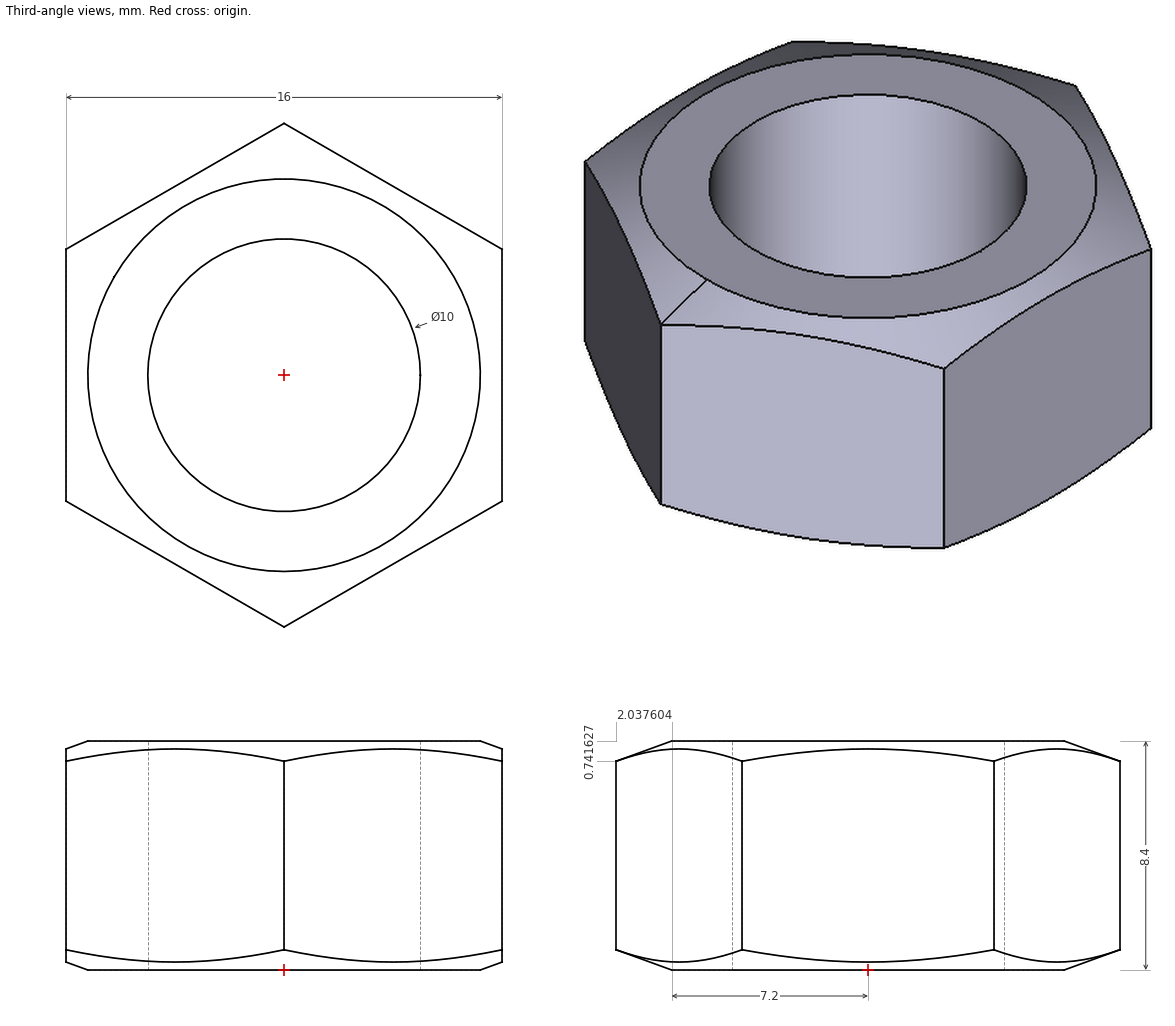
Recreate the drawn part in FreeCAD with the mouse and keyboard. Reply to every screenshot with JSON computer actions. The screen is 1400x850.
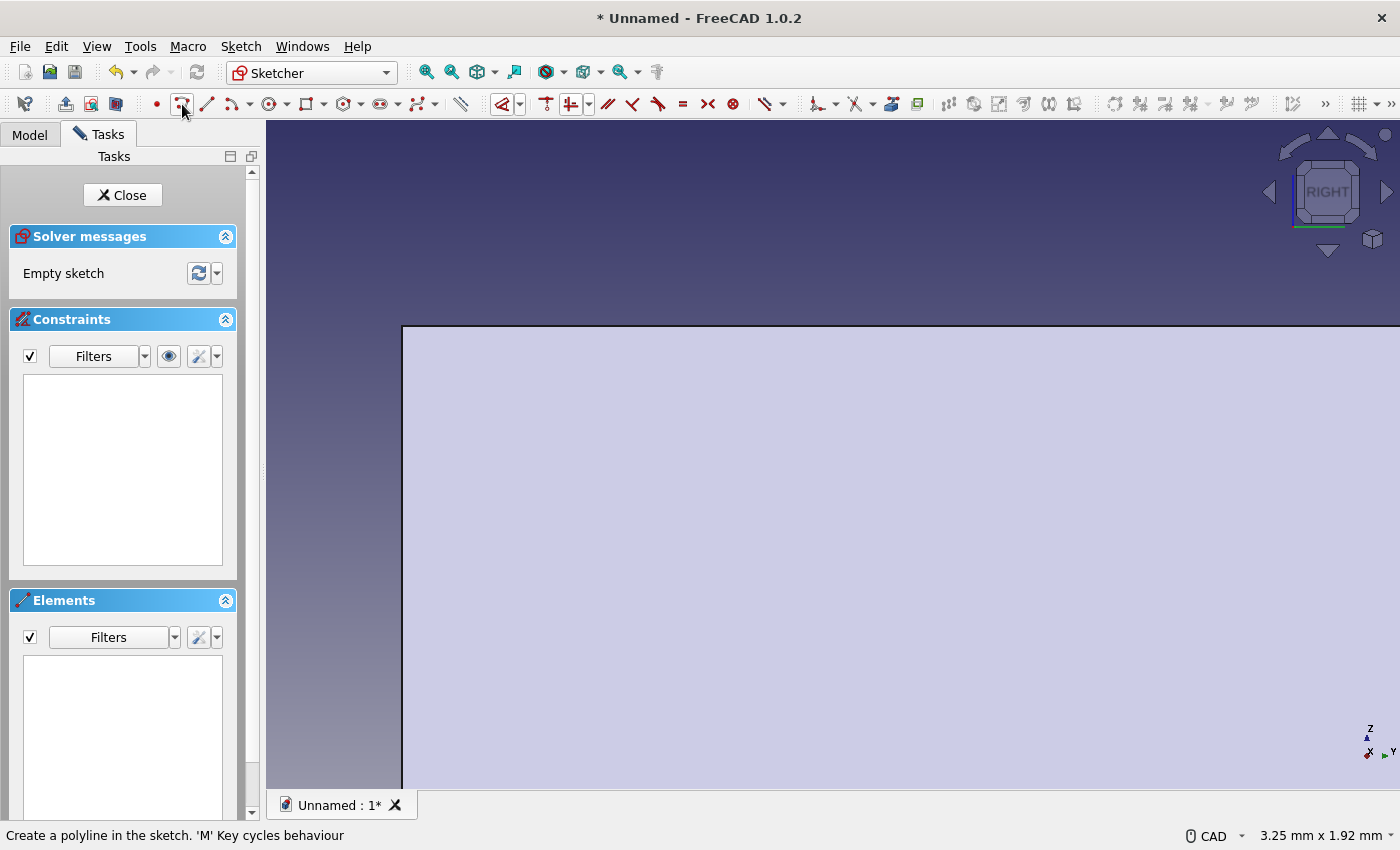
{"action": "left_click", "coordinate": [1112, 326]}
{"action": "left_click", "coordinate": [402, 326]}
{"action": "left_click", "coordinate": [402, 585]}
{"action": "left_click", "coordinate": [1112, 327]}
{"action": "key", "text": "Escape"}
{"action": "key", "text": "Escape"}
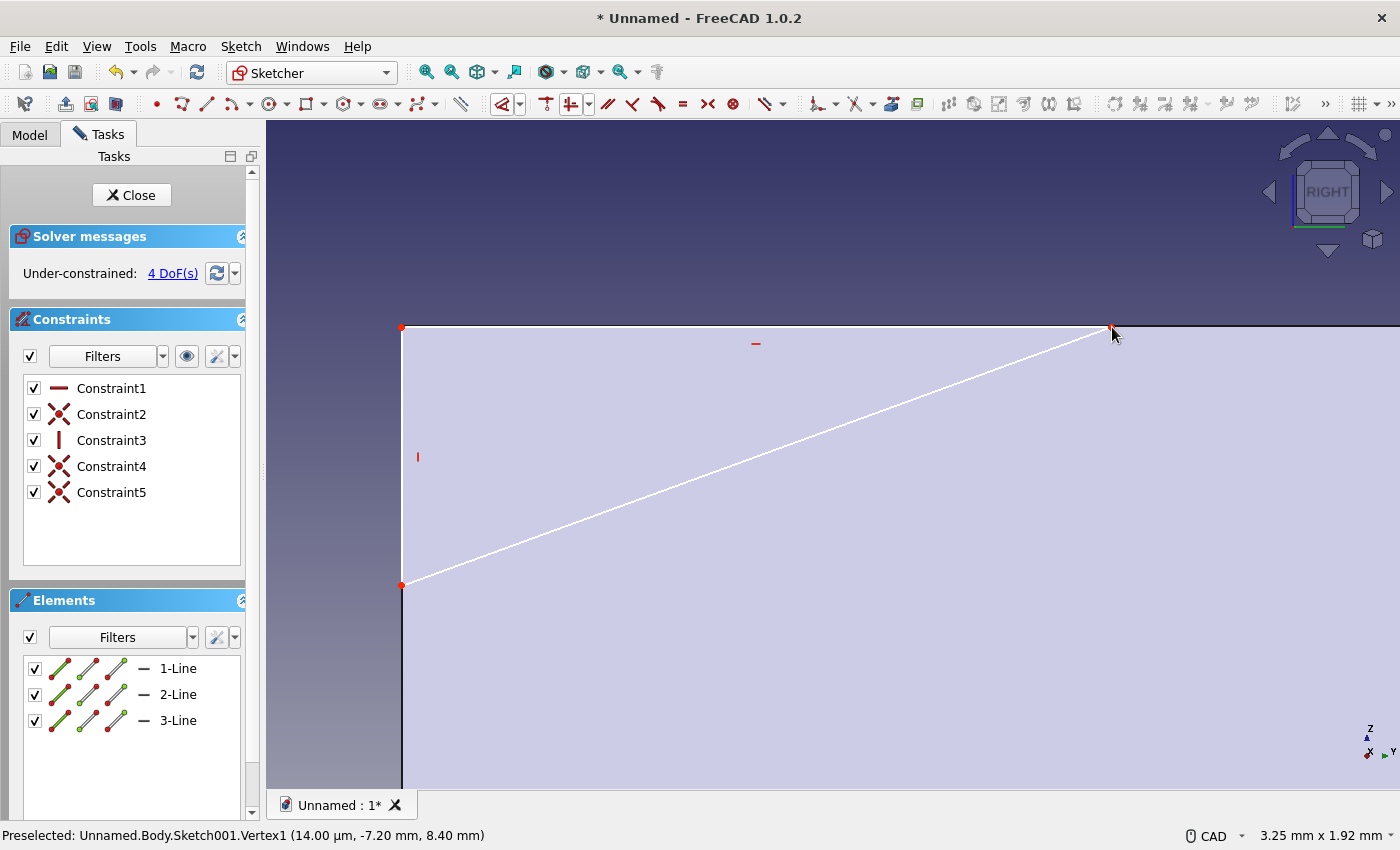
{"action": "left_click", "coordinate": [1112, 327]}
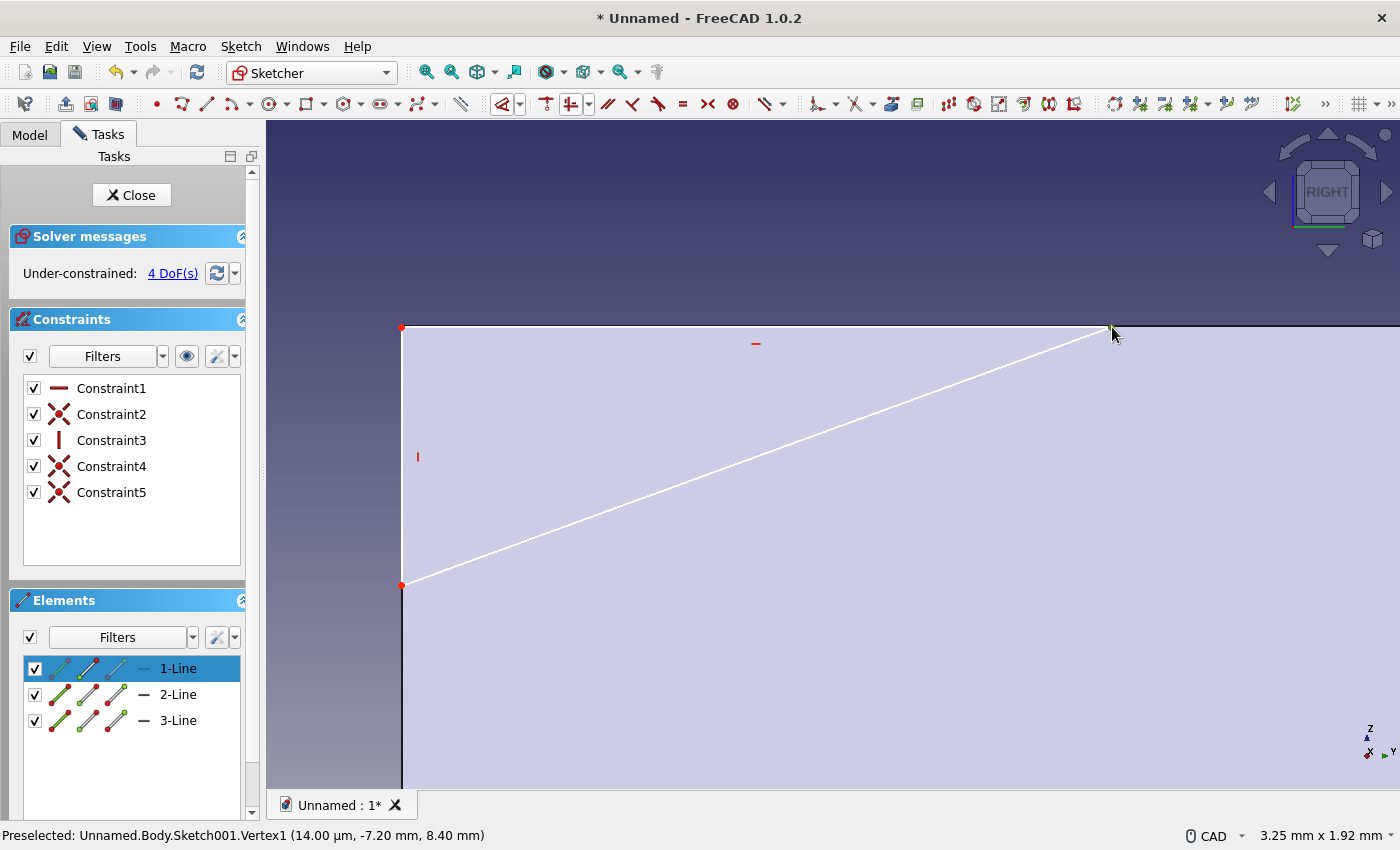
{"action": "key", "text": "l"}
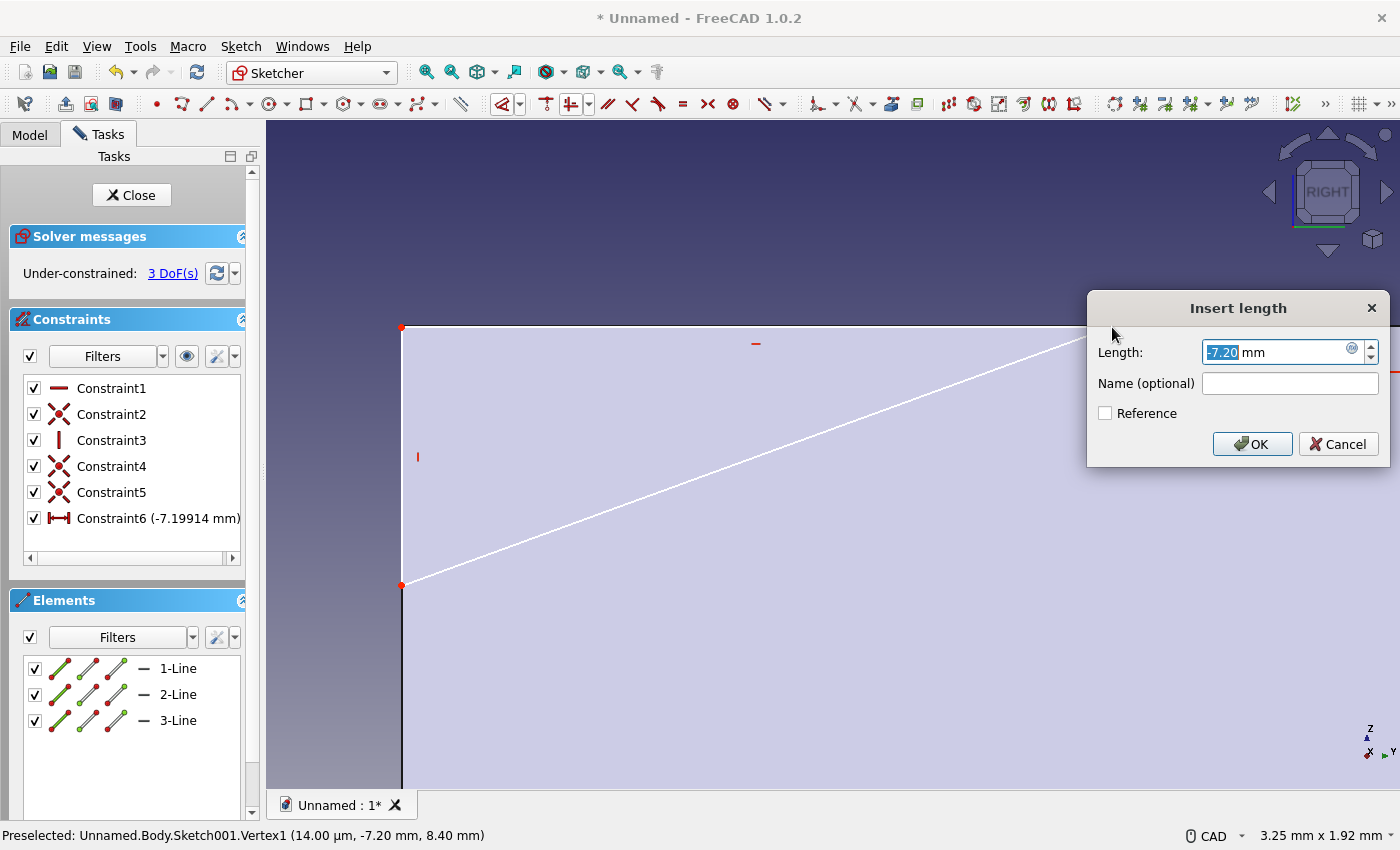
{"action": "type", "text": "-7.2"}
{"action": "key", "text": "Return"}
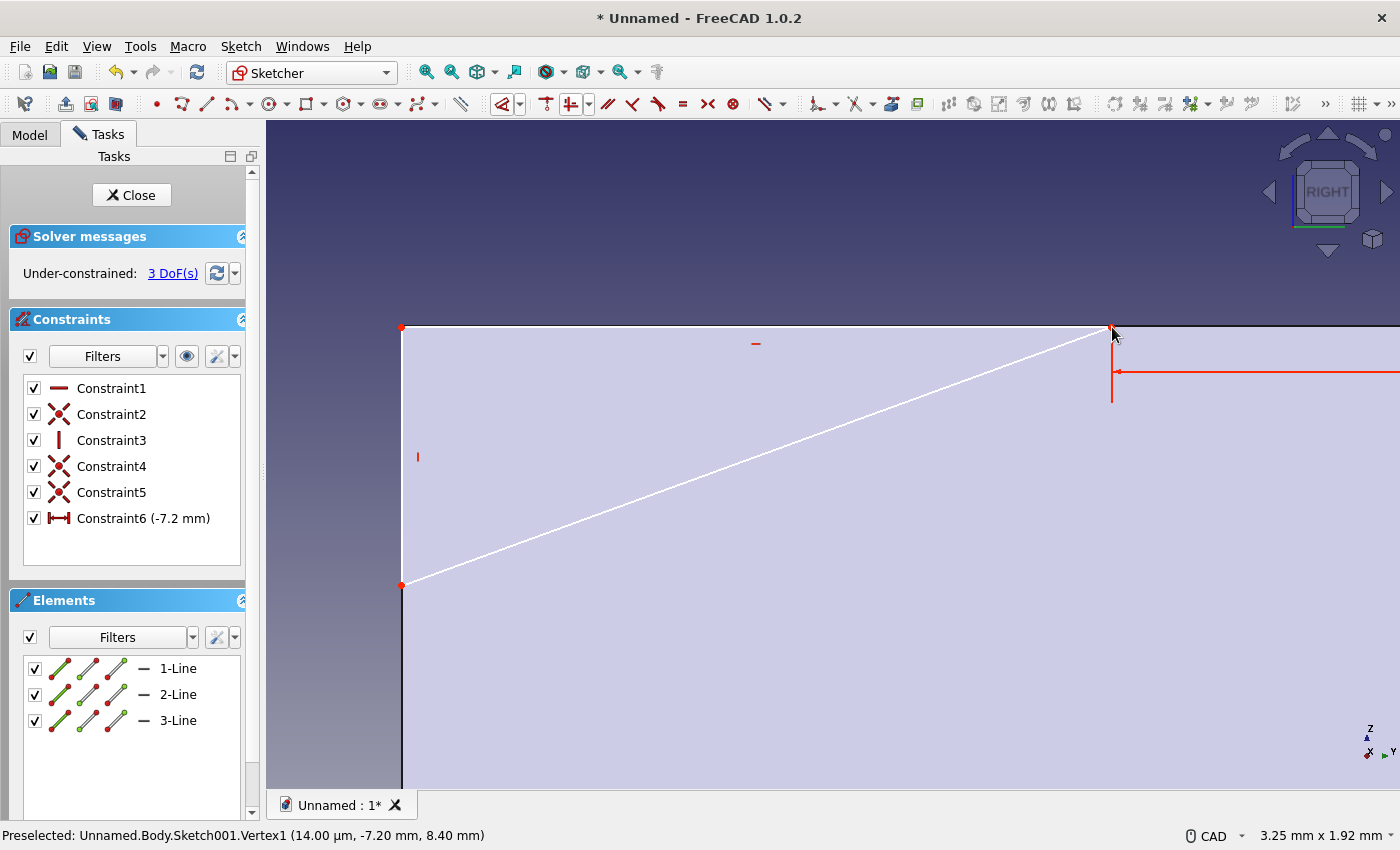
{"action": "left_click", "coordinate": [1112, 327]}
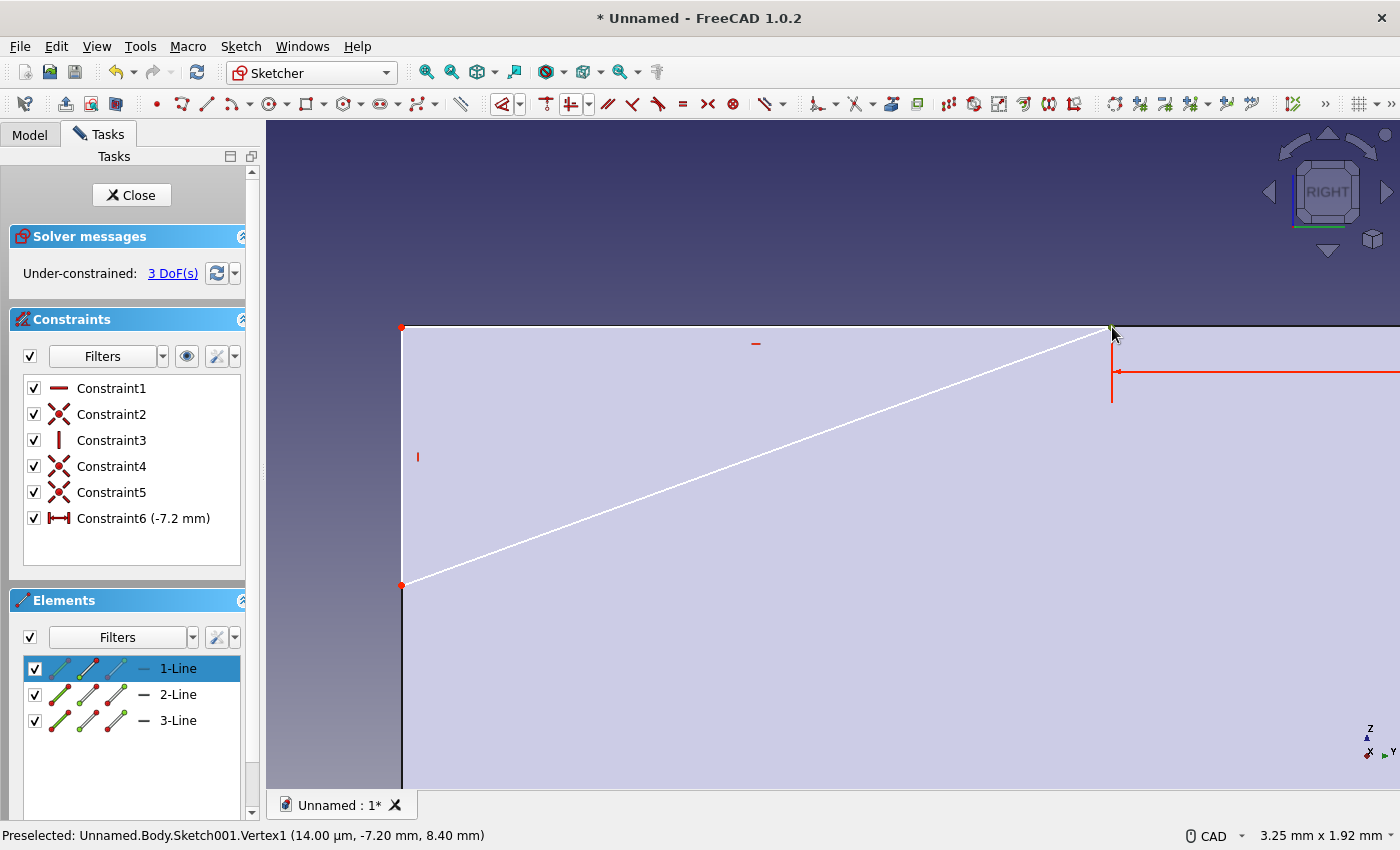
{"action": "left_click", "coordinate": [520, 104]}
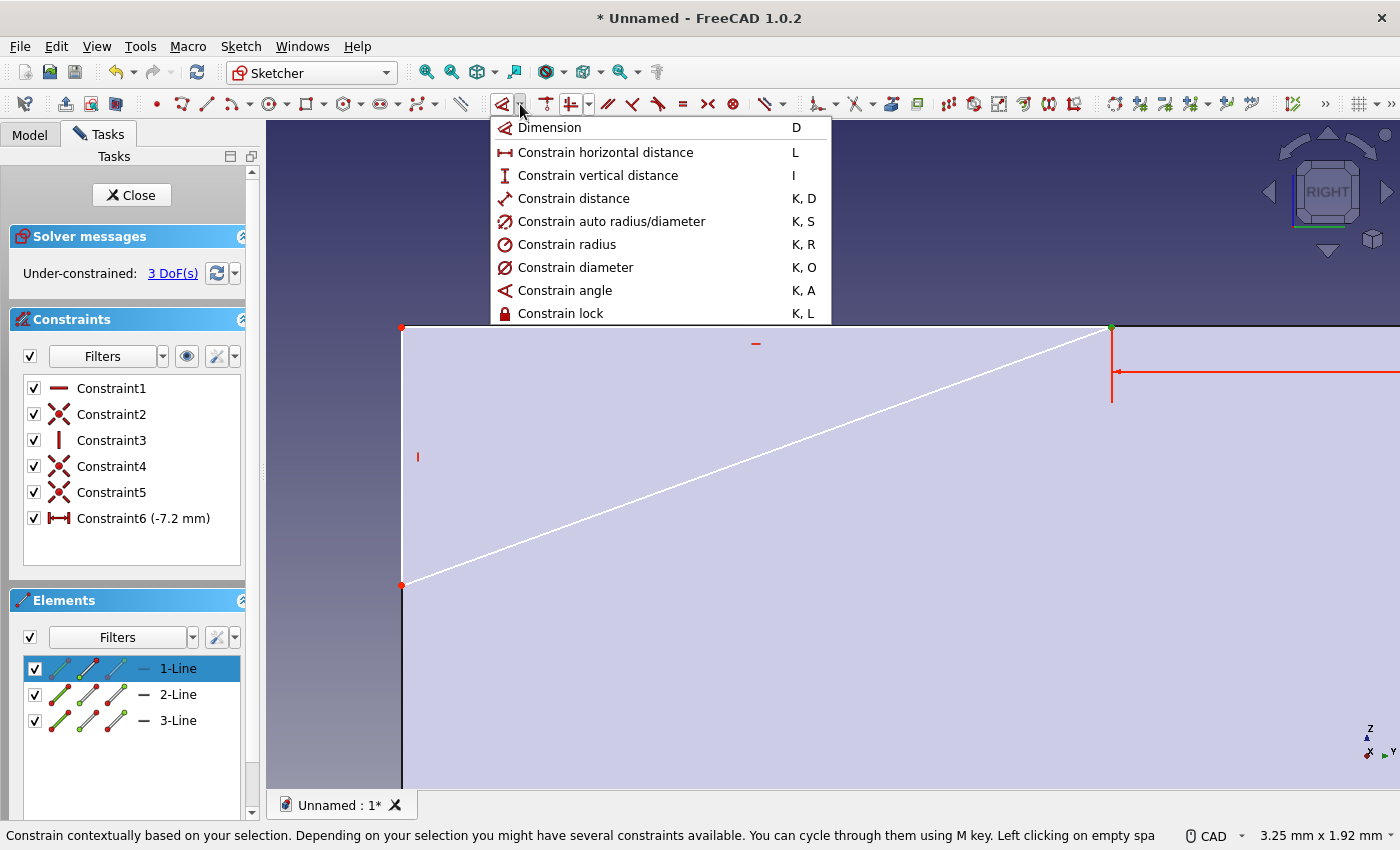
{"action": "left_click", "coordinate": [661, 176]}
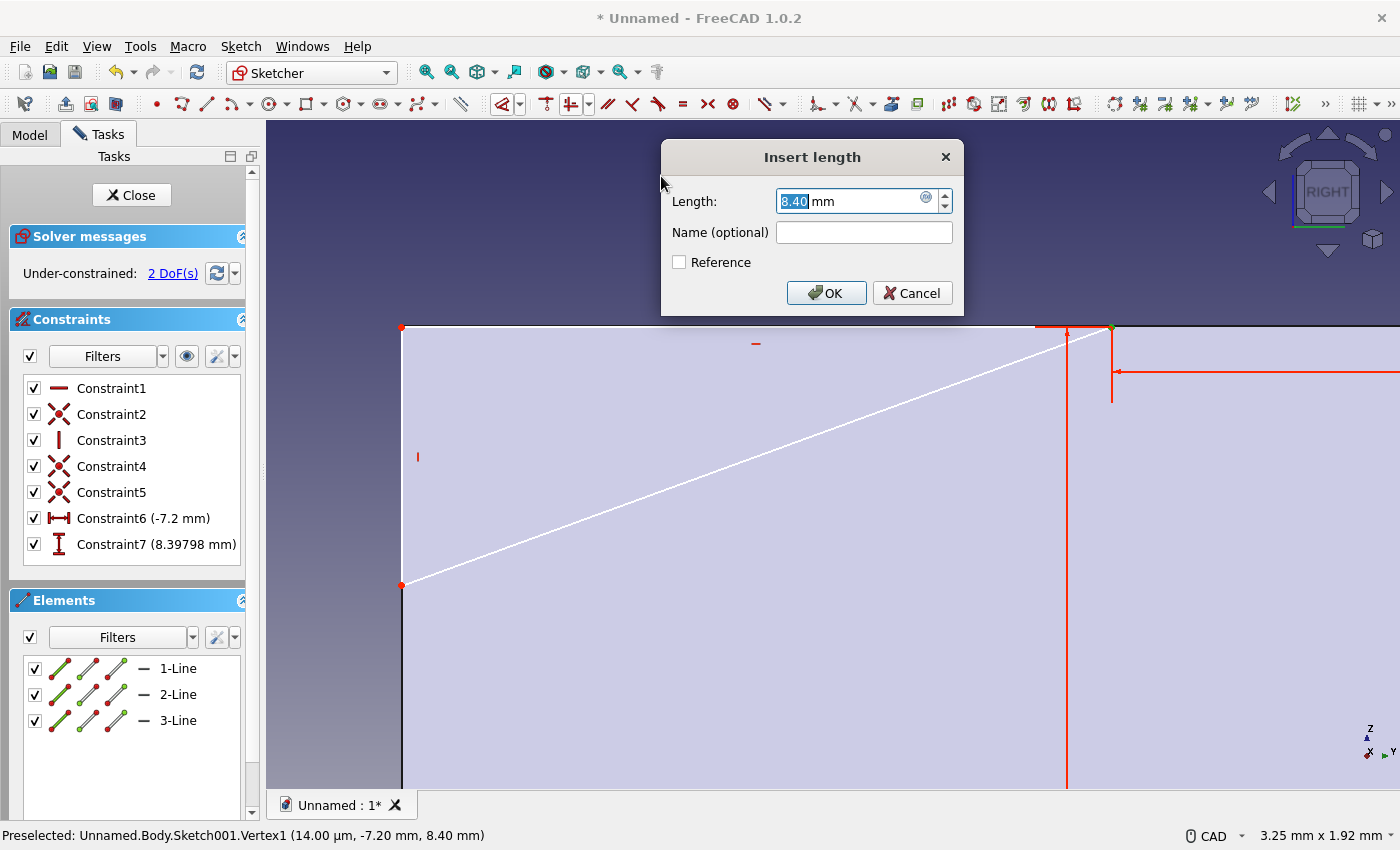
{"action": "type", "text": "8.4"}
{"action": "key", "text": "Return"}